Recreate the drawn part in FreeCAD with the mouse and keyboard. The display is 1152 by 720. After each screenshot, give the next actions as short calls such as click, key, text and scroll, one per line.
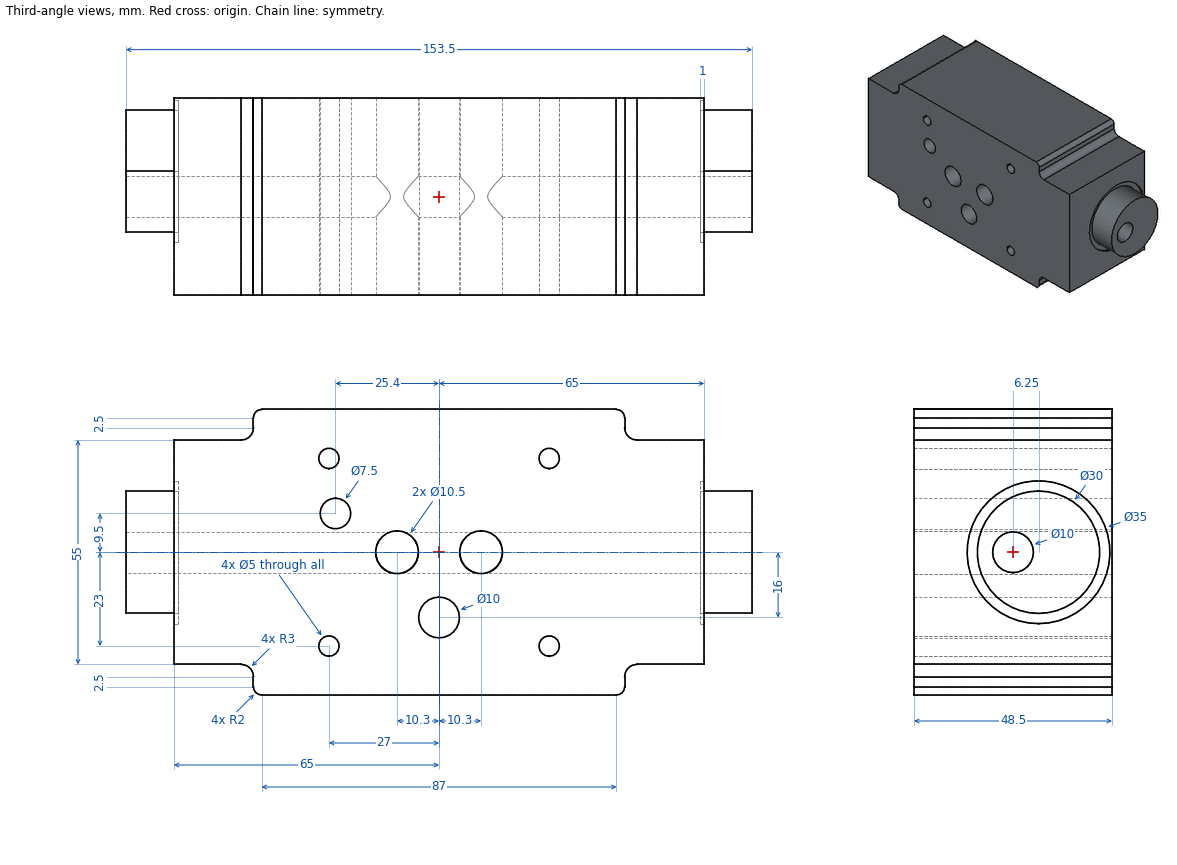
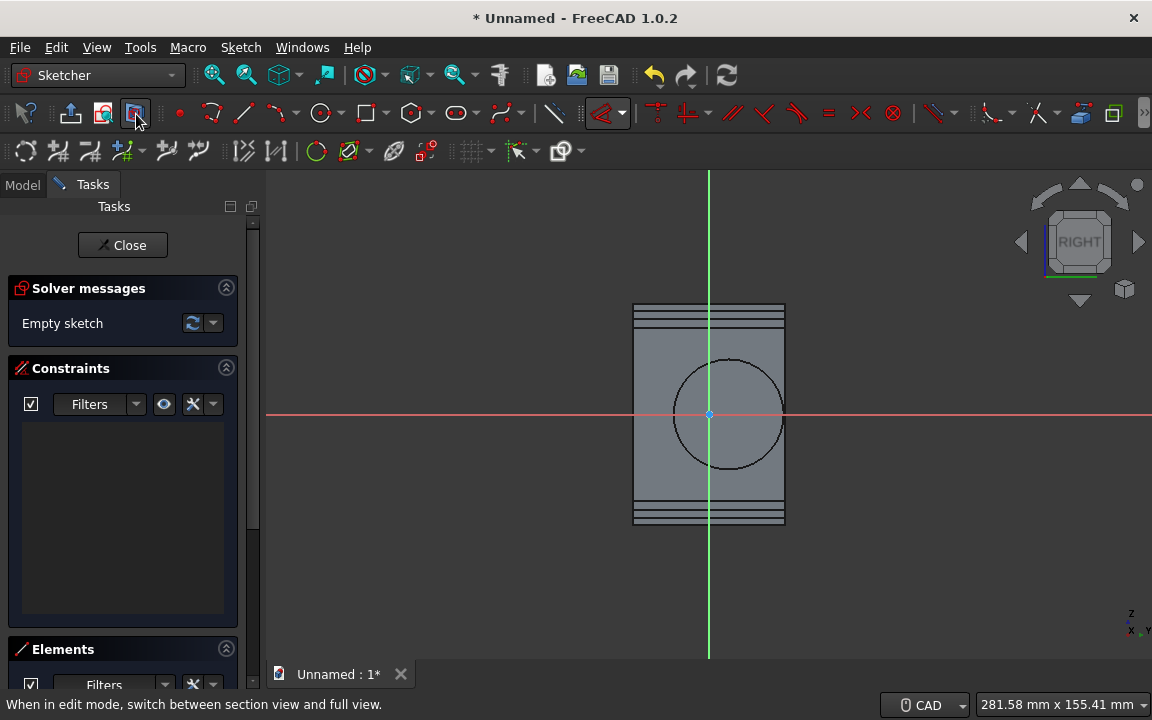
scroll(767, 415, up, 6)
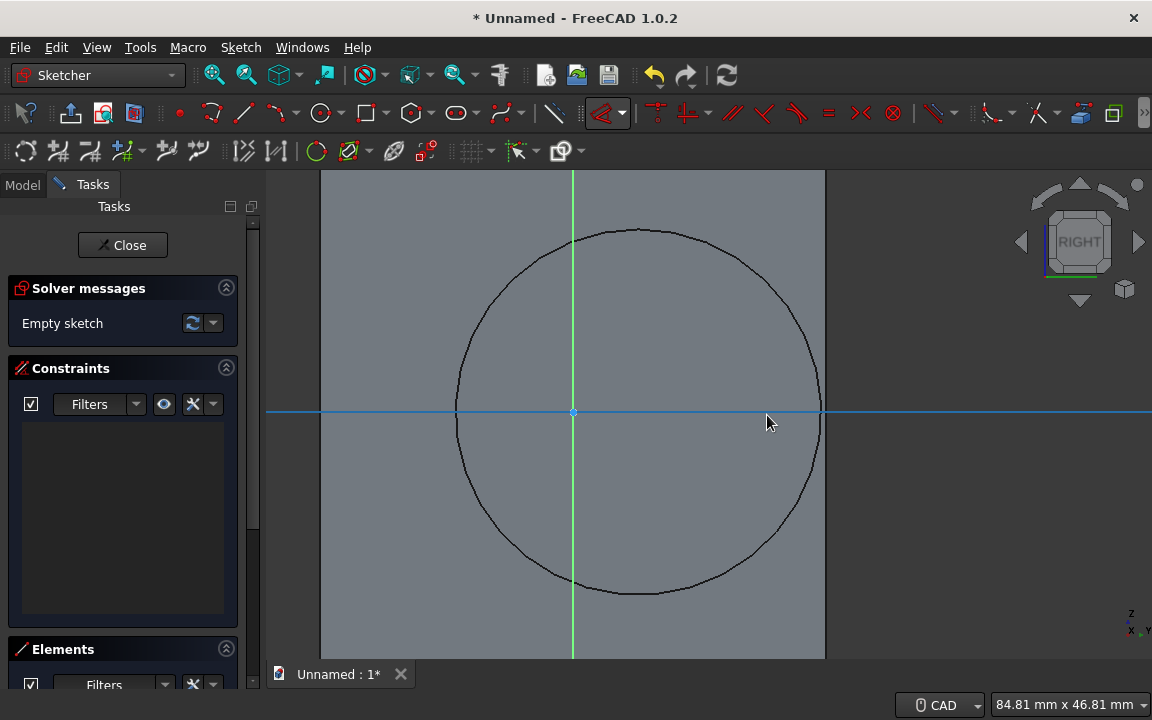
click(322, 114)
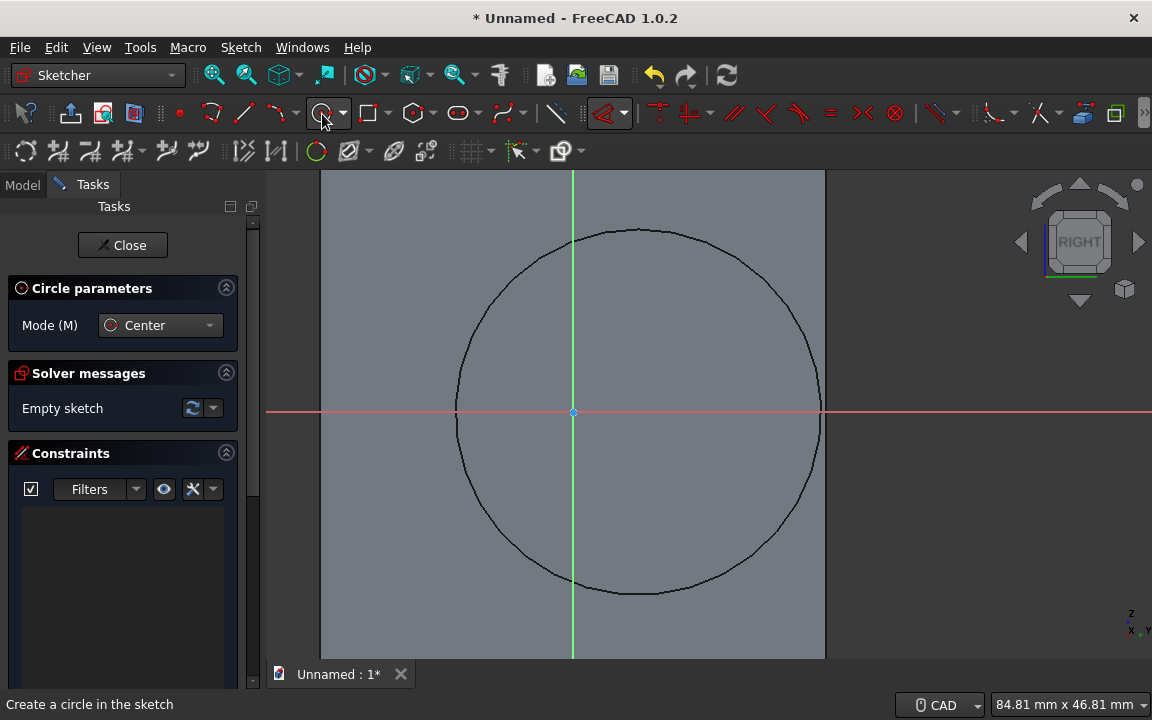
click(638, 412)
move(749, 301)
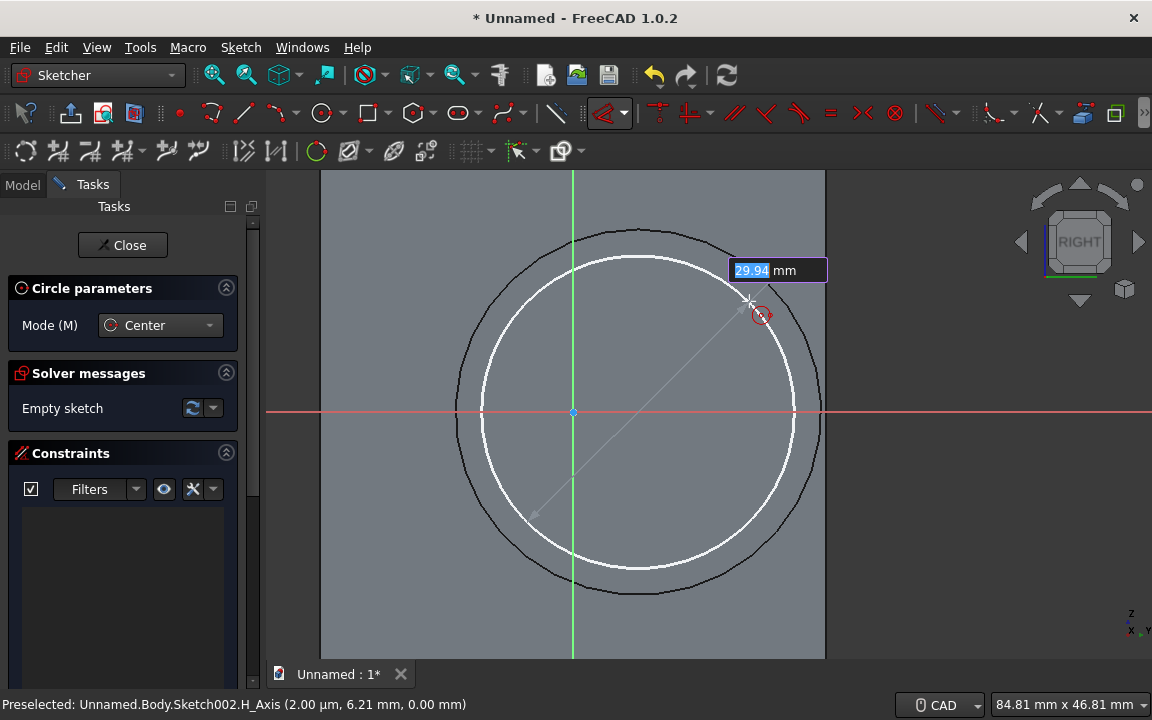
text(30)
key(Return)
key(Escape)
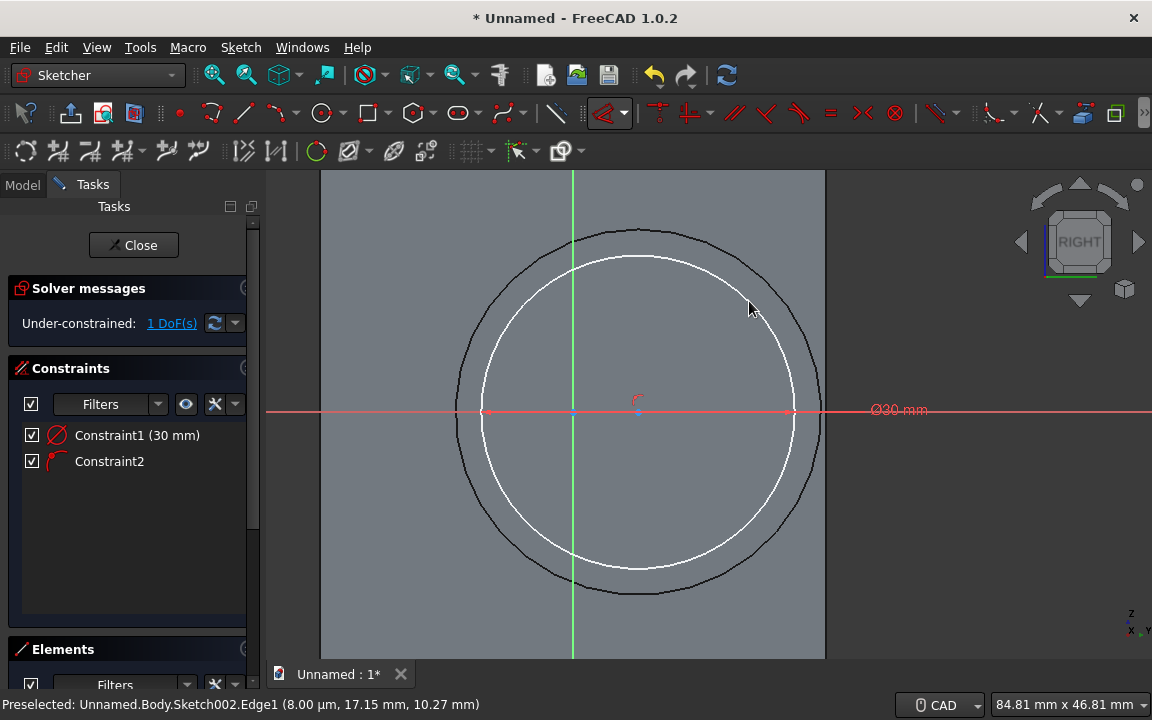
click(638, 412)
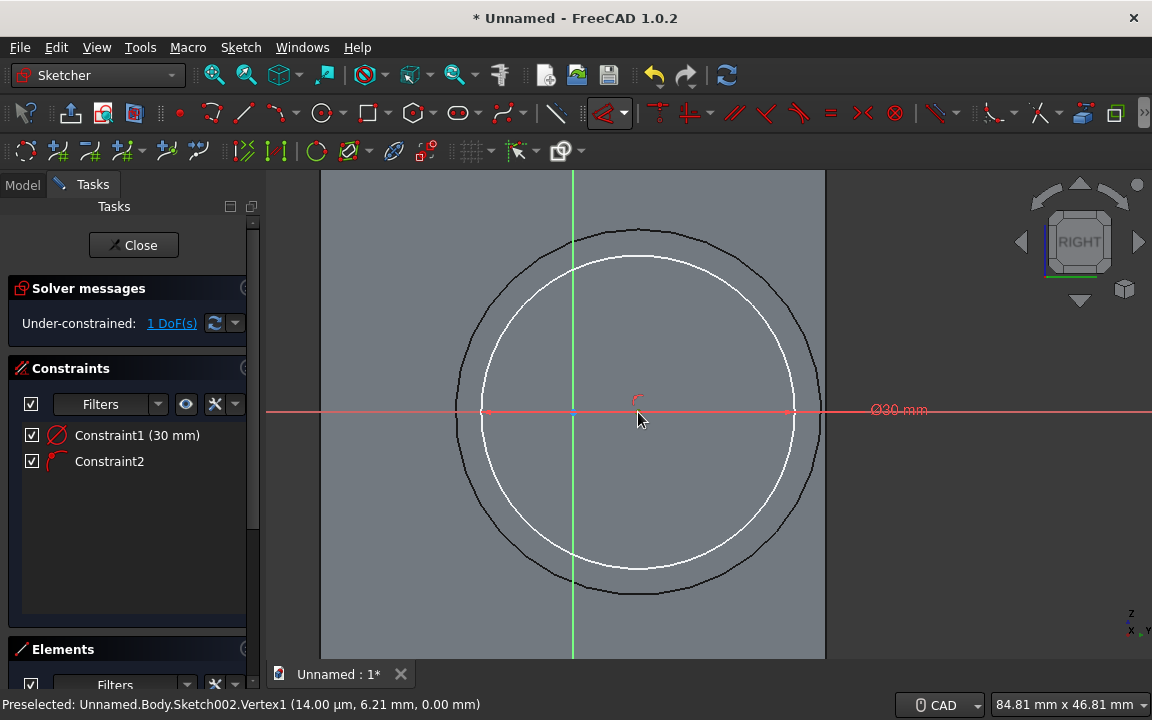
click(626, 114)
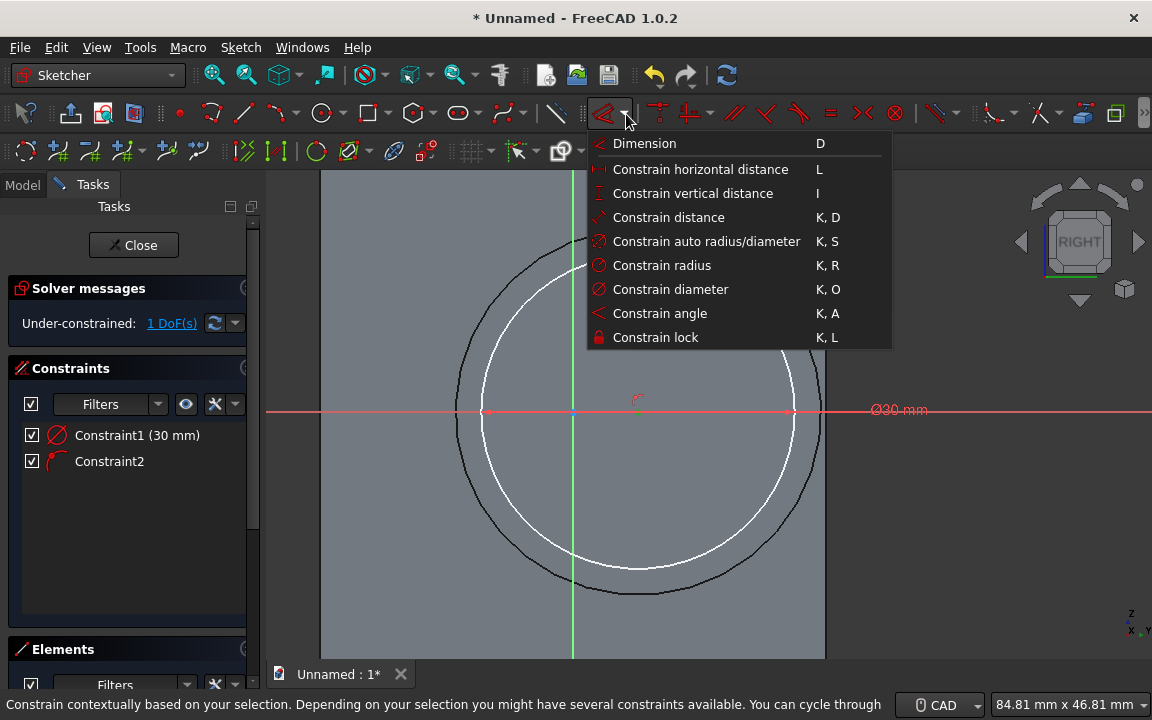
click(740, 169)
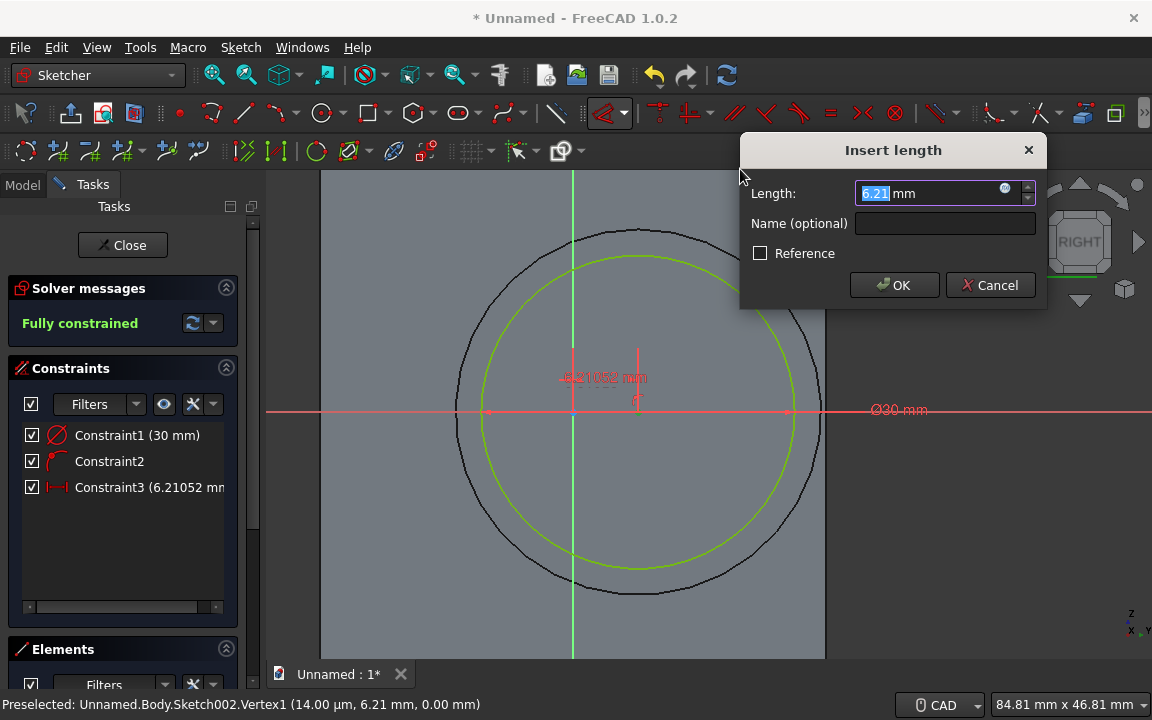
text(6.25)
key(Return)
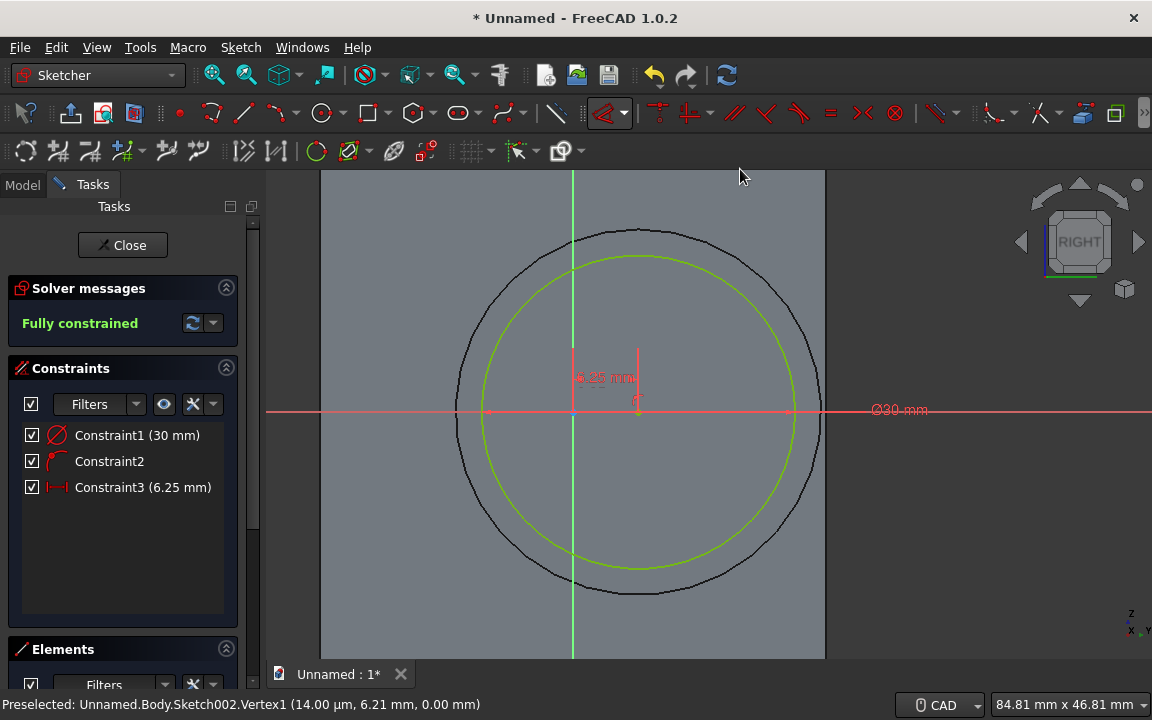
click(123, 245)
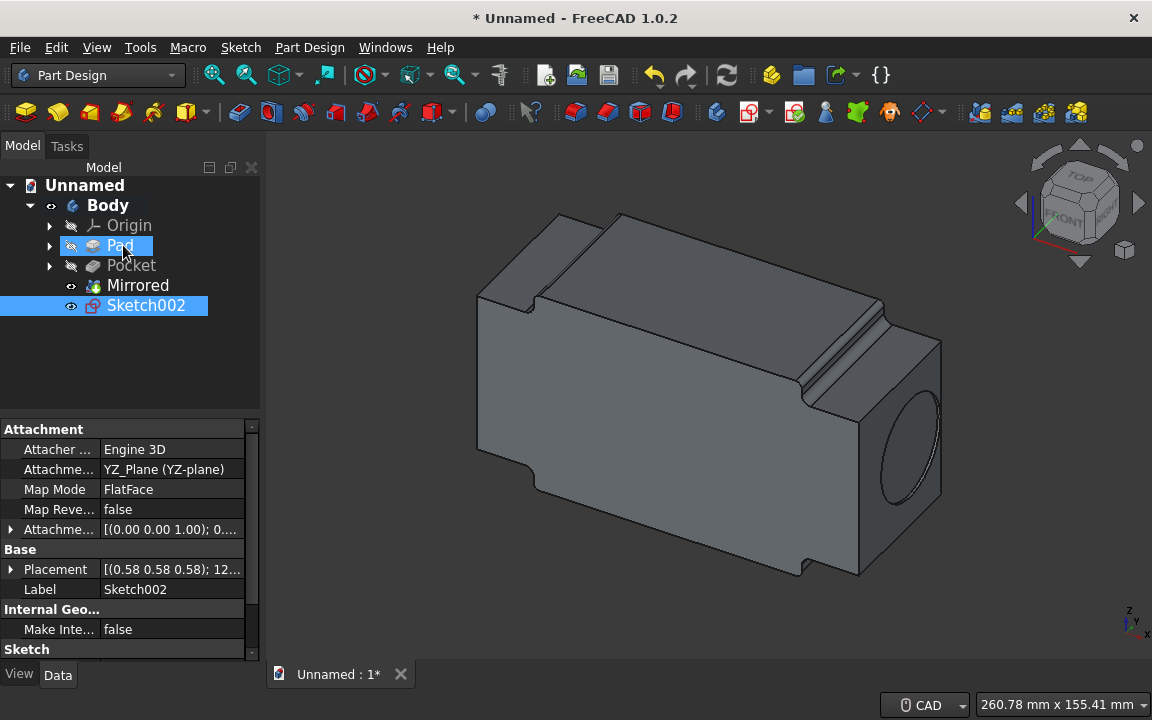
click(26, 112)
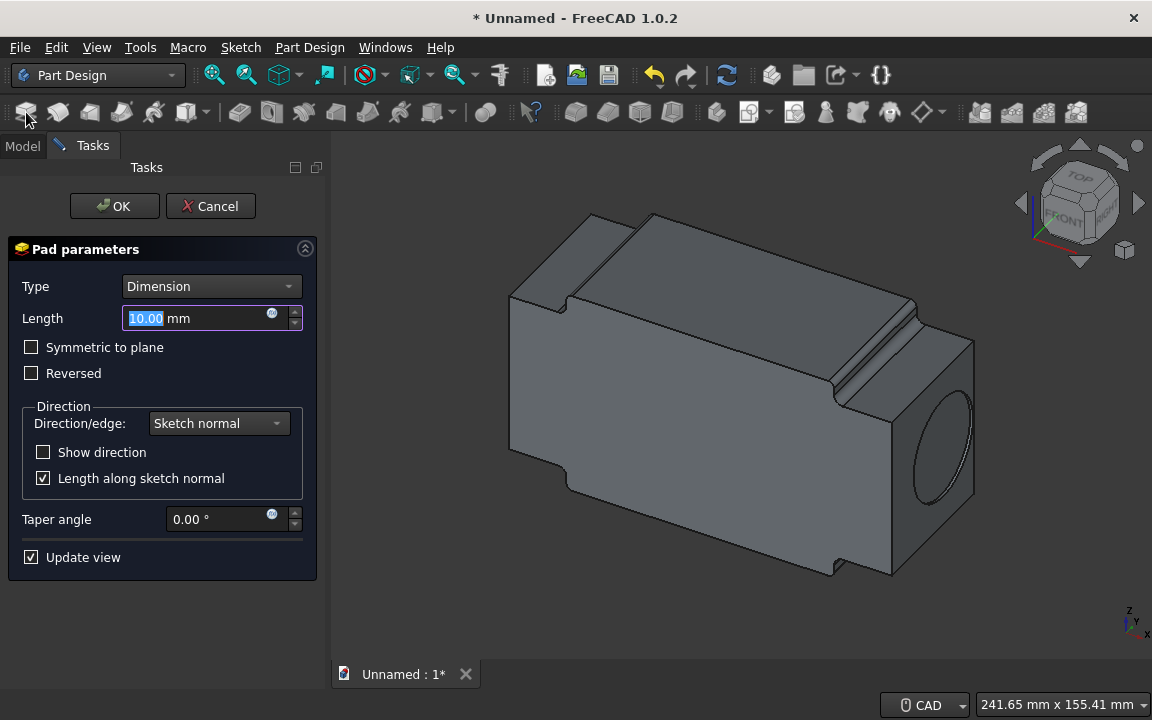
text(153.5)
key(Tab)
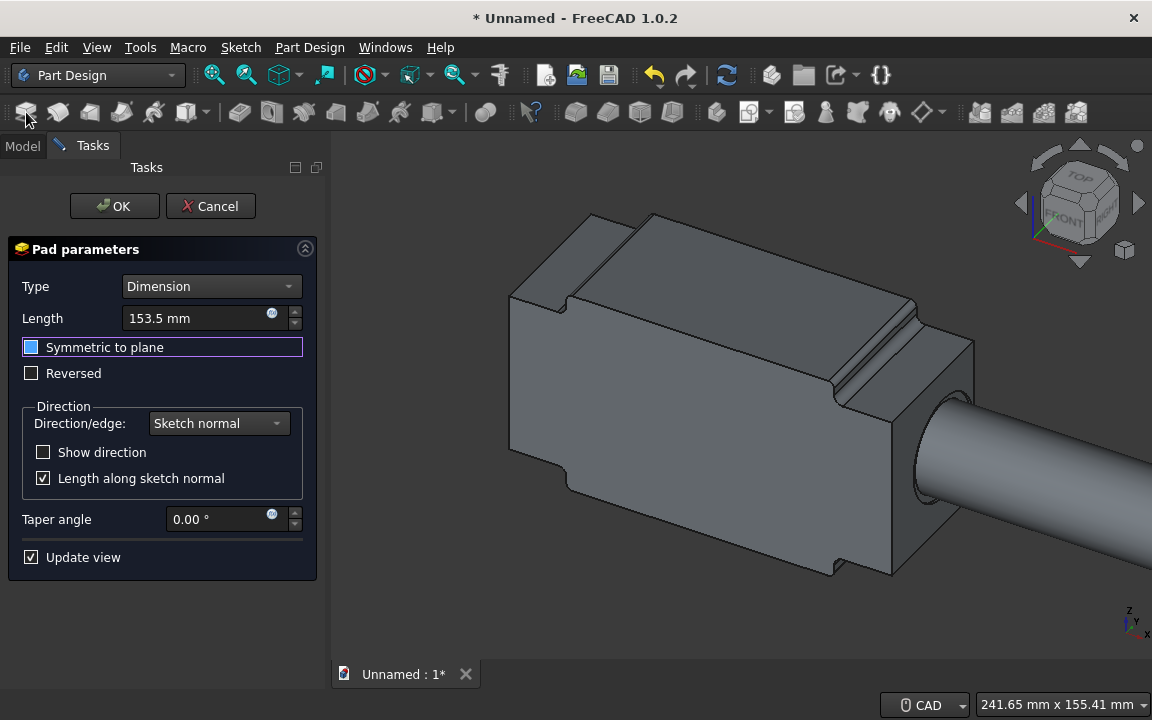
click(30, 347)